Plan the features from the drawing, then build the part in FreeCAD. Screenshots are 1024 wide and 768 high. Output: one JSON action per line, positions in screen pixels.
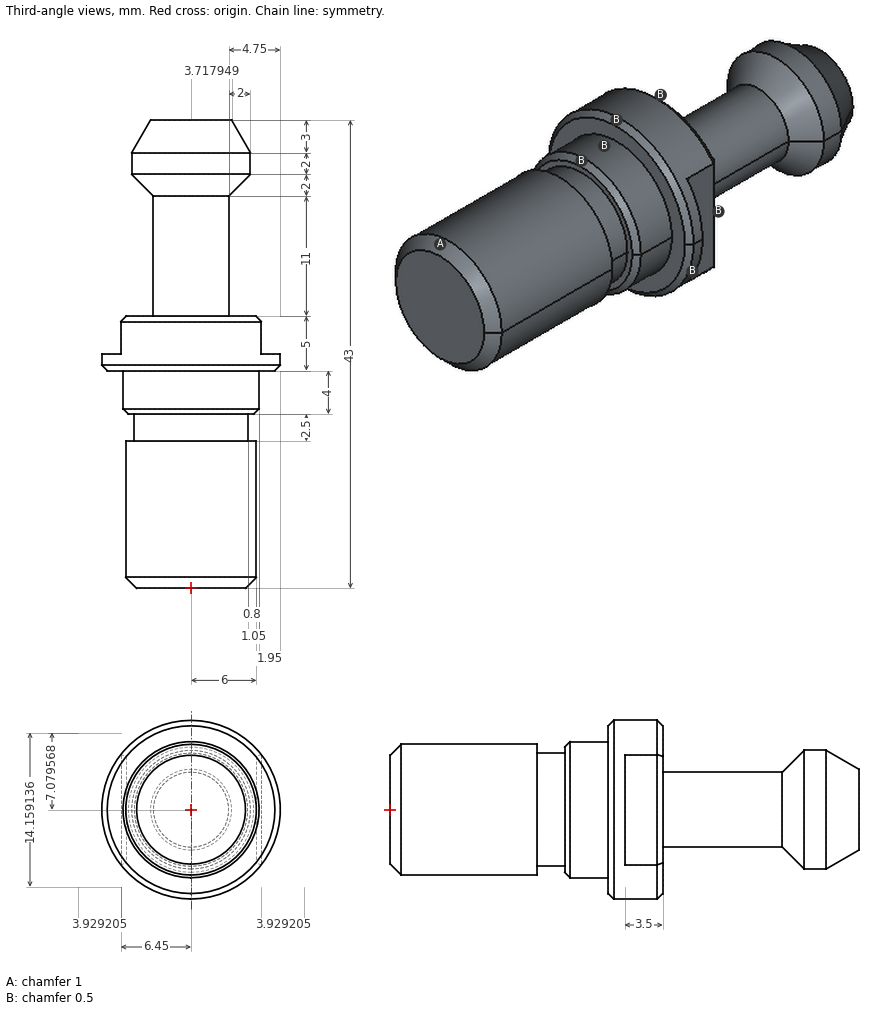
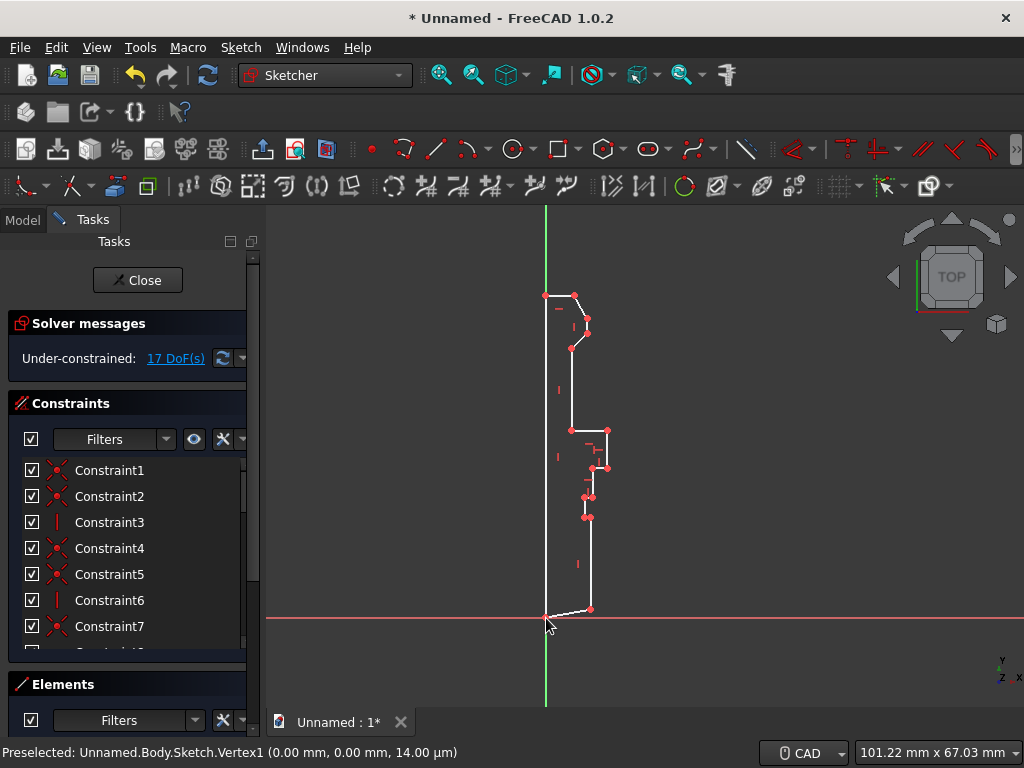
{"action": "left_click", "coordinate": [559, 615]}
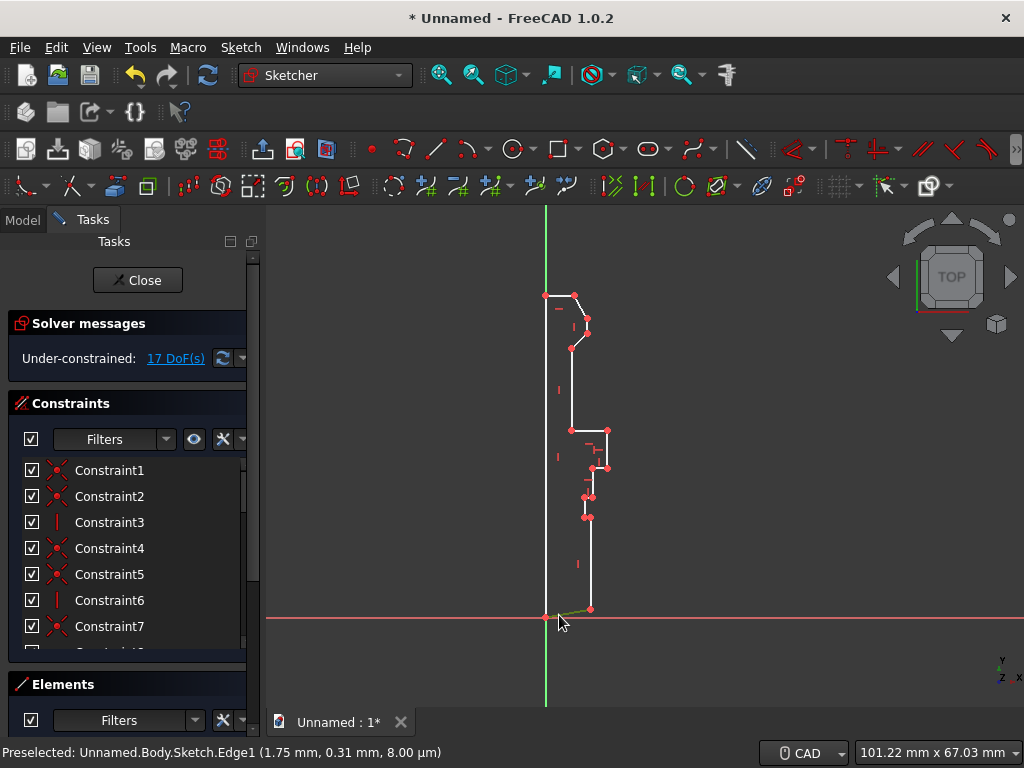
{"action": "key", "text": "h"}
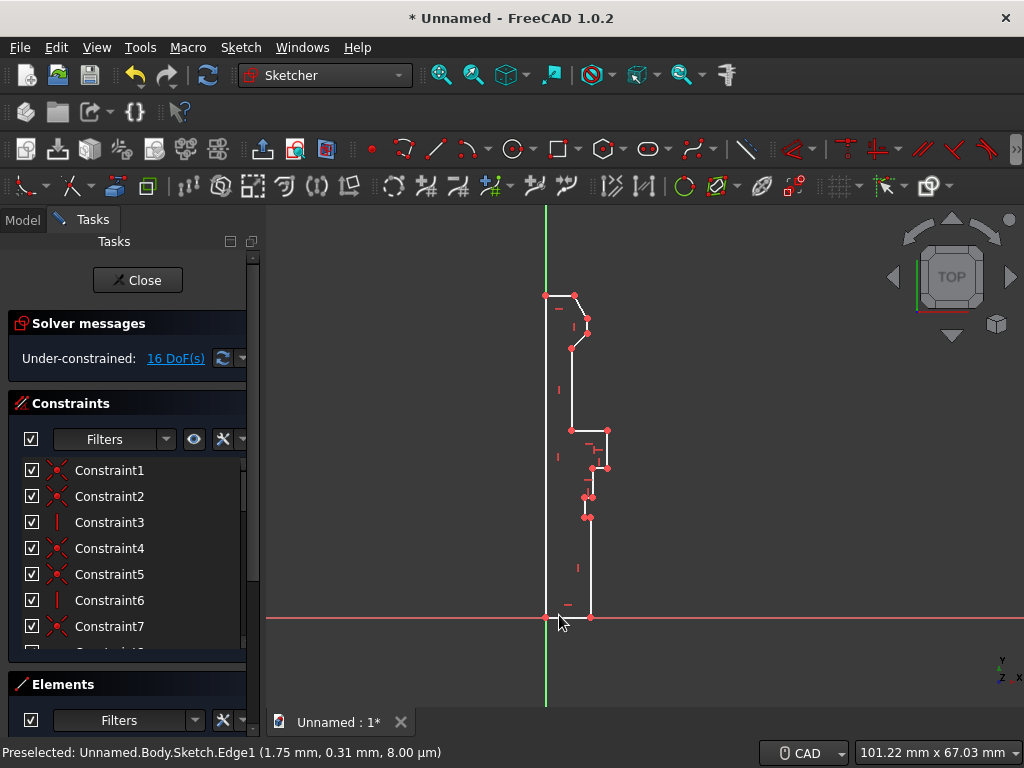
{"action": "scroll", "coordinate": [588, 517], "scroll_direction": "up", "scroll_amount": 8}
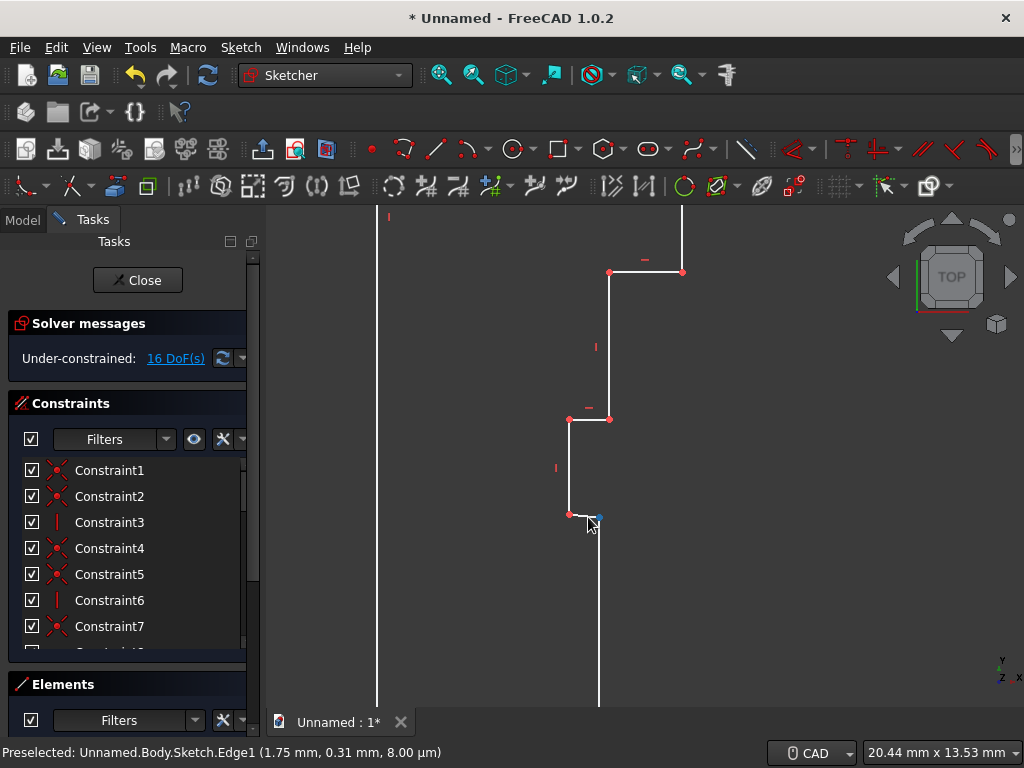
{"action": "left_click", "coordinate": [584, 516]}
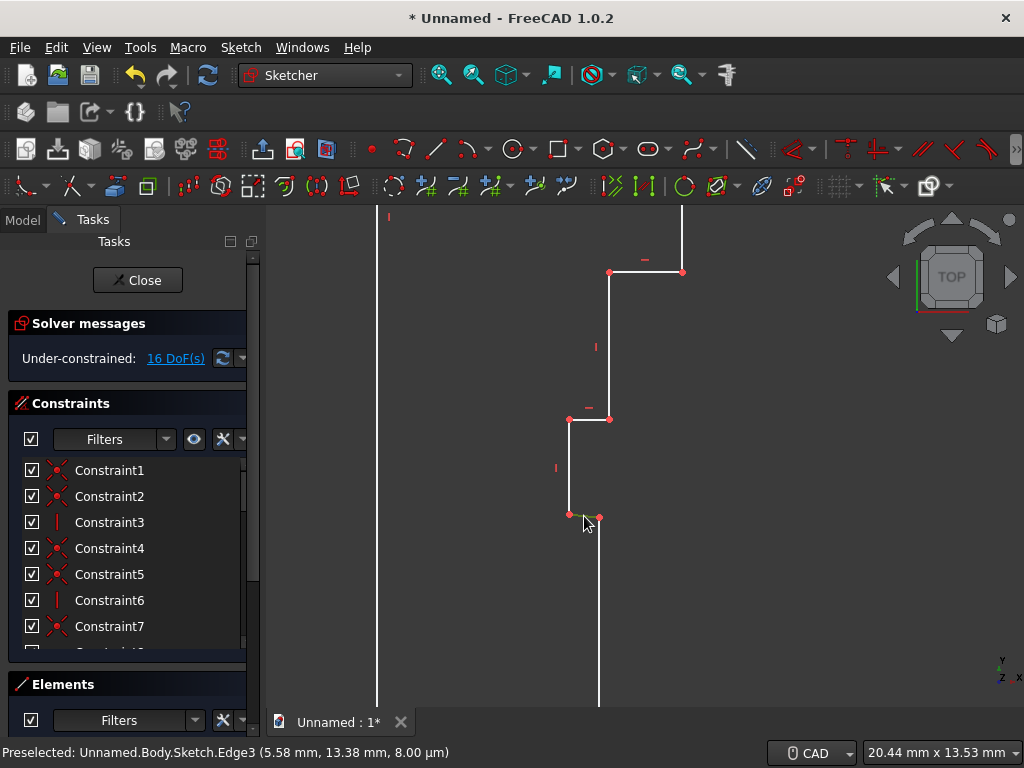
{"action": "left_click", "coordinate": [900, 150]}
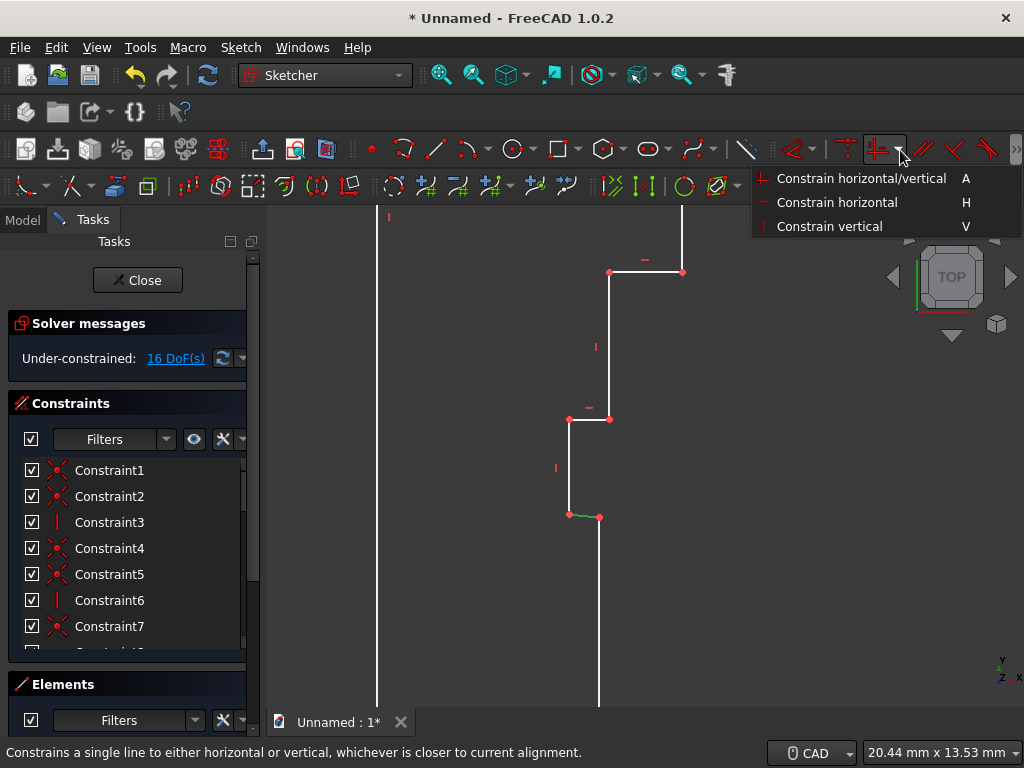
{"action": "left_click", "coordinate": [887, 202]}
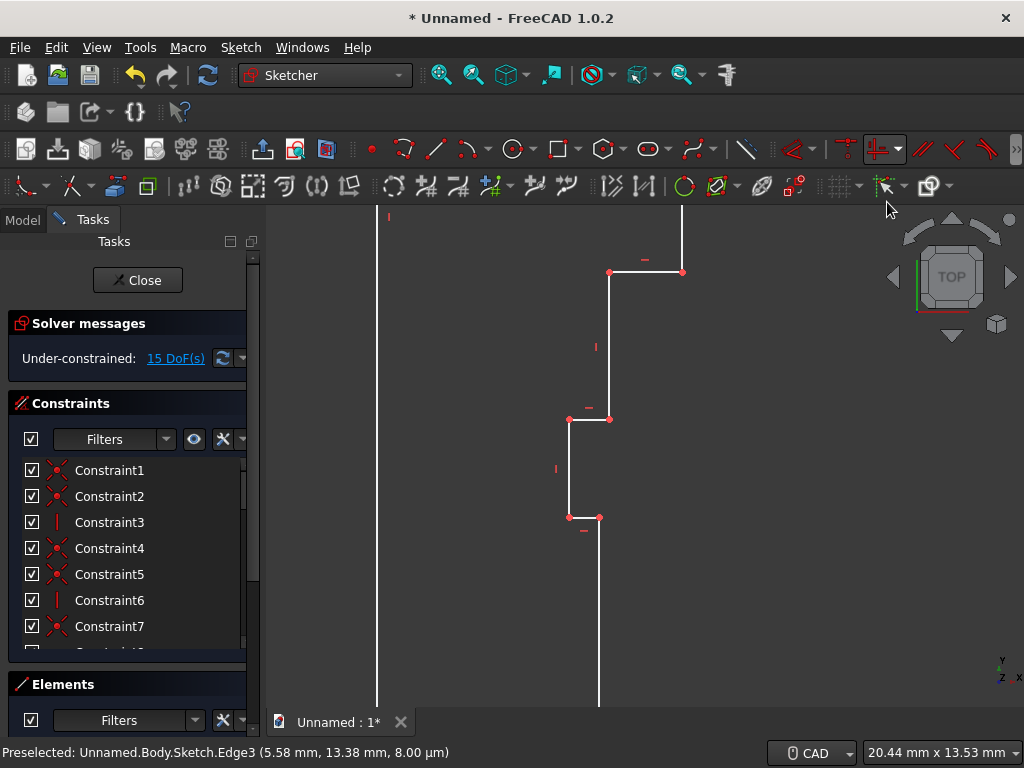
{"action": "left_click", "coordinate": [792, 150]}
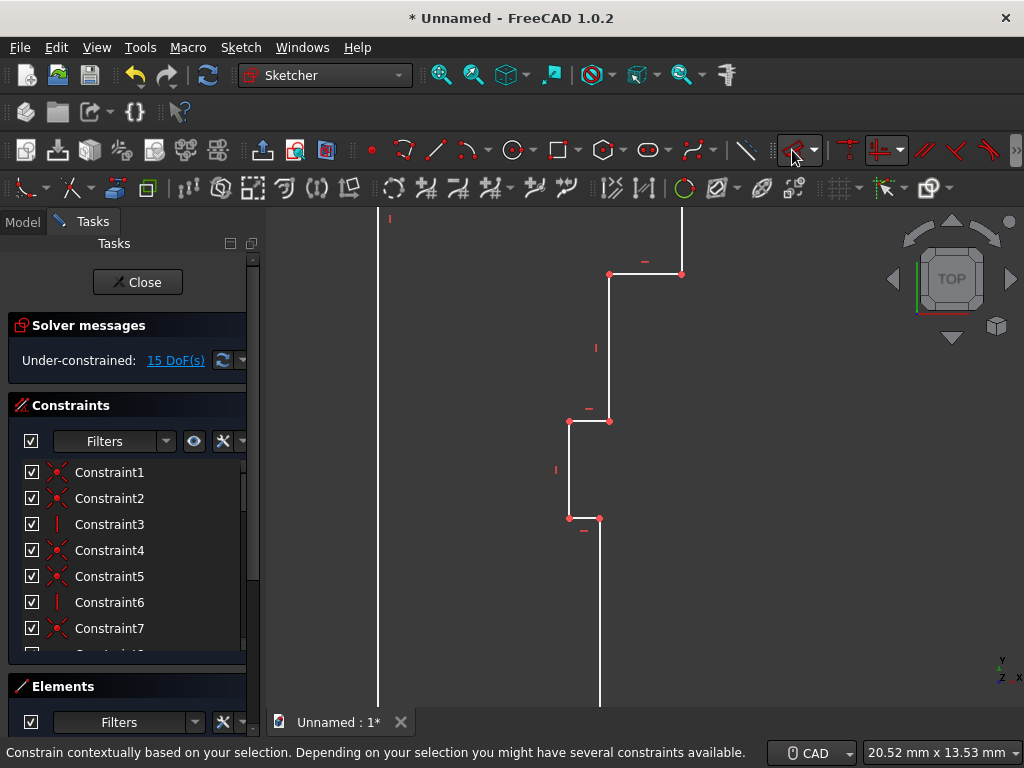
{"action": "scroll", "coordinate": [588, 518], "scroll_direction": "down", "scroll_amount": 8}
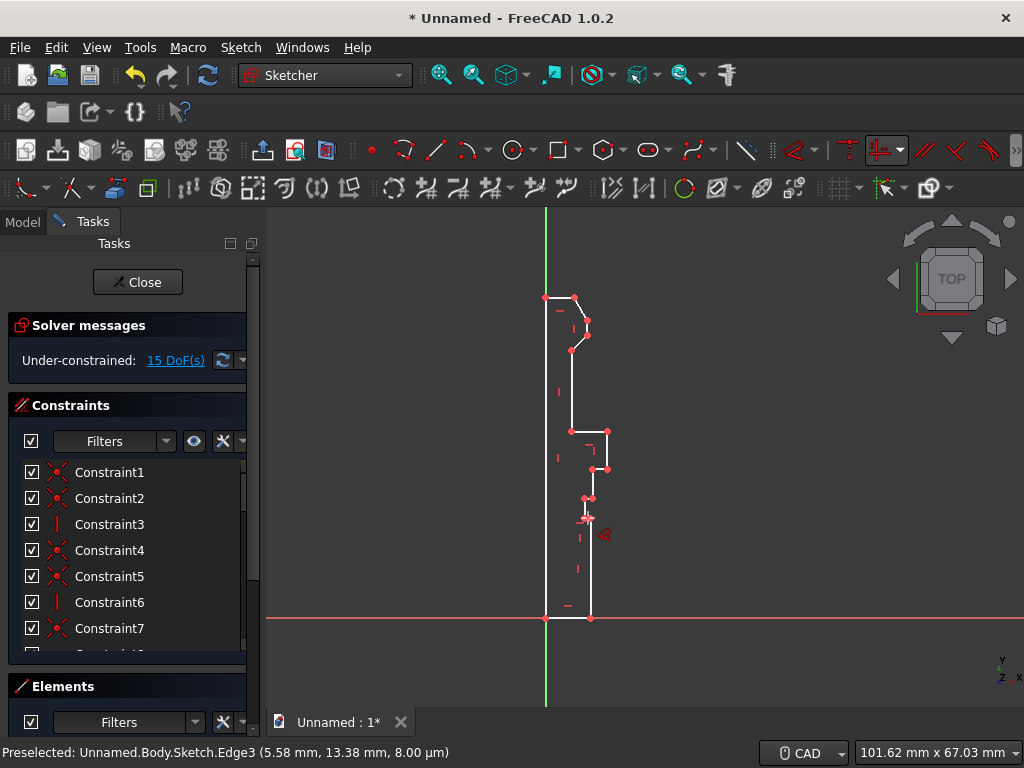
{"action": "left_click", "coordinate": [559, 618]}
{"action": "left_click", "coordinate": [568, 652]}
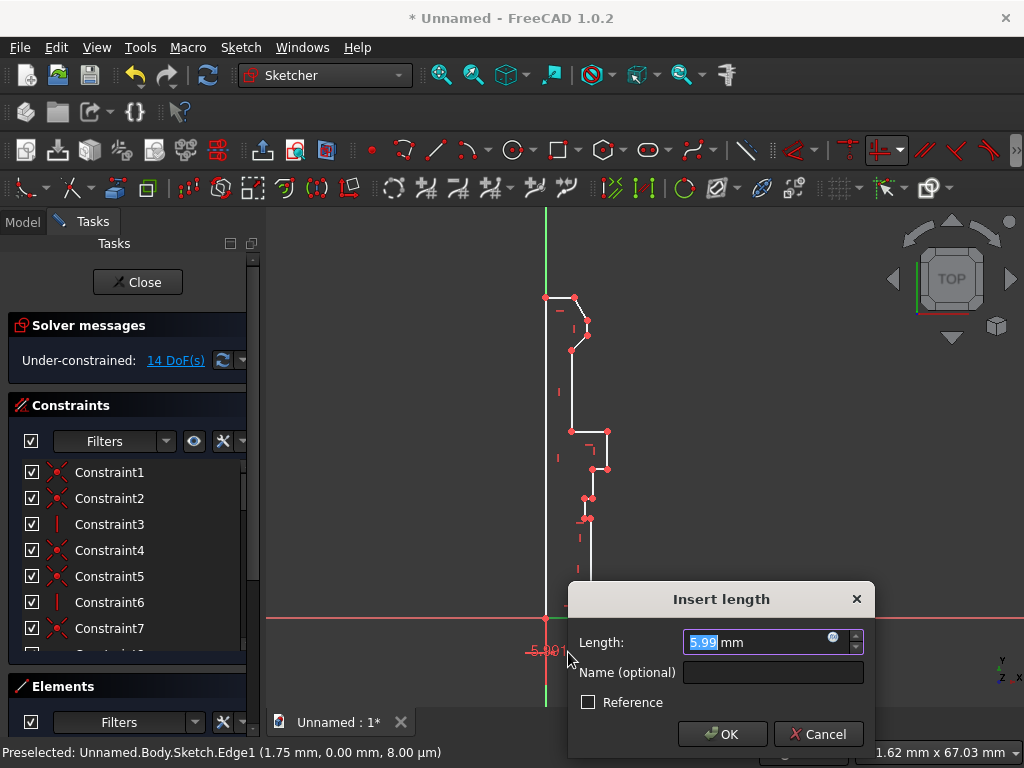
{"action": "type", "text": "6"}
{"action": "key", "text": "Return"}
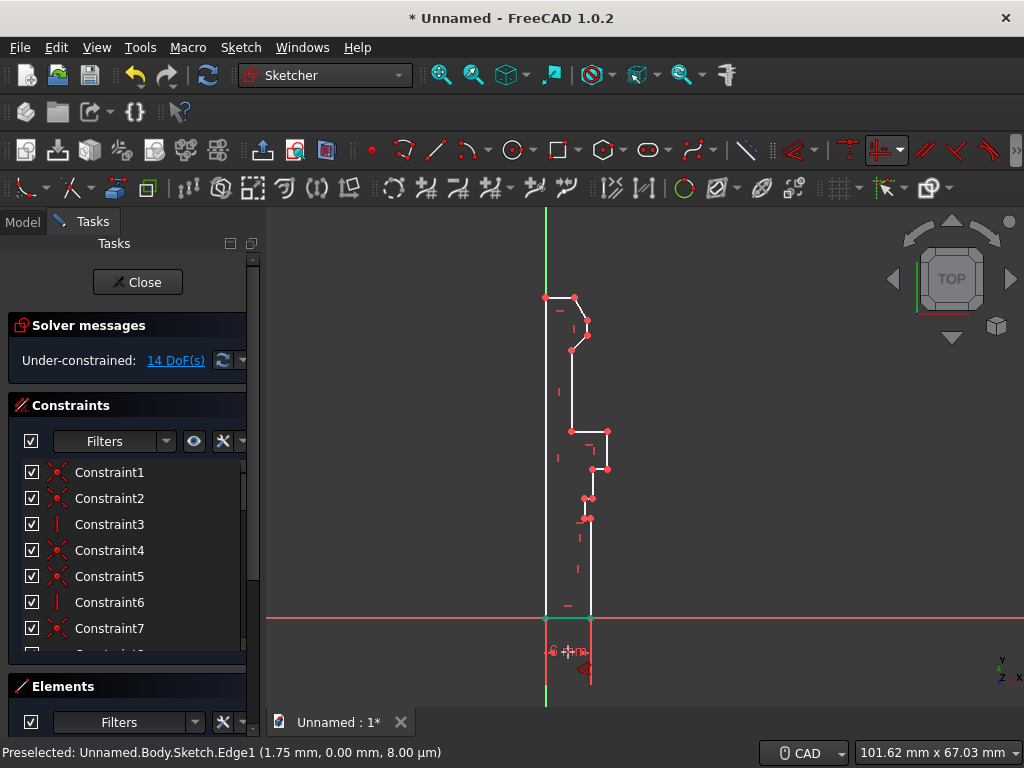
{"action": "scroll", "coordinate": [593, 487], "scroll_direction": "up", "scroll_amount": 2}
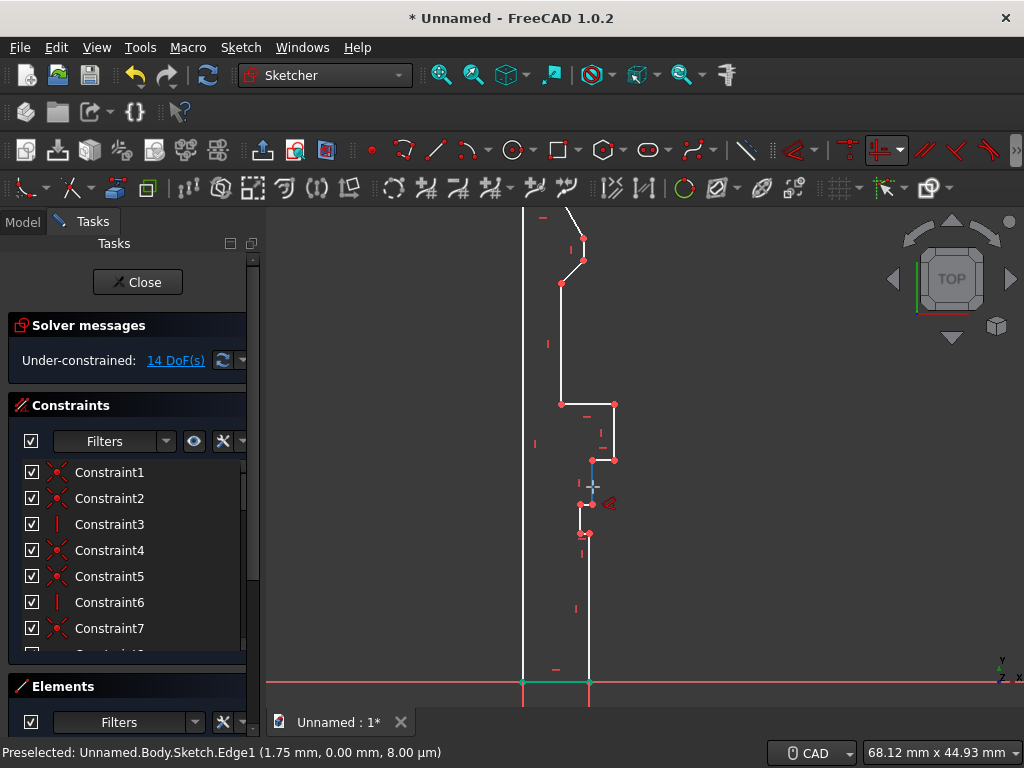
{"action": "left_click", "coordinate": [592, 487]}
{"action": "left_click", "coordinate": [626, 482]}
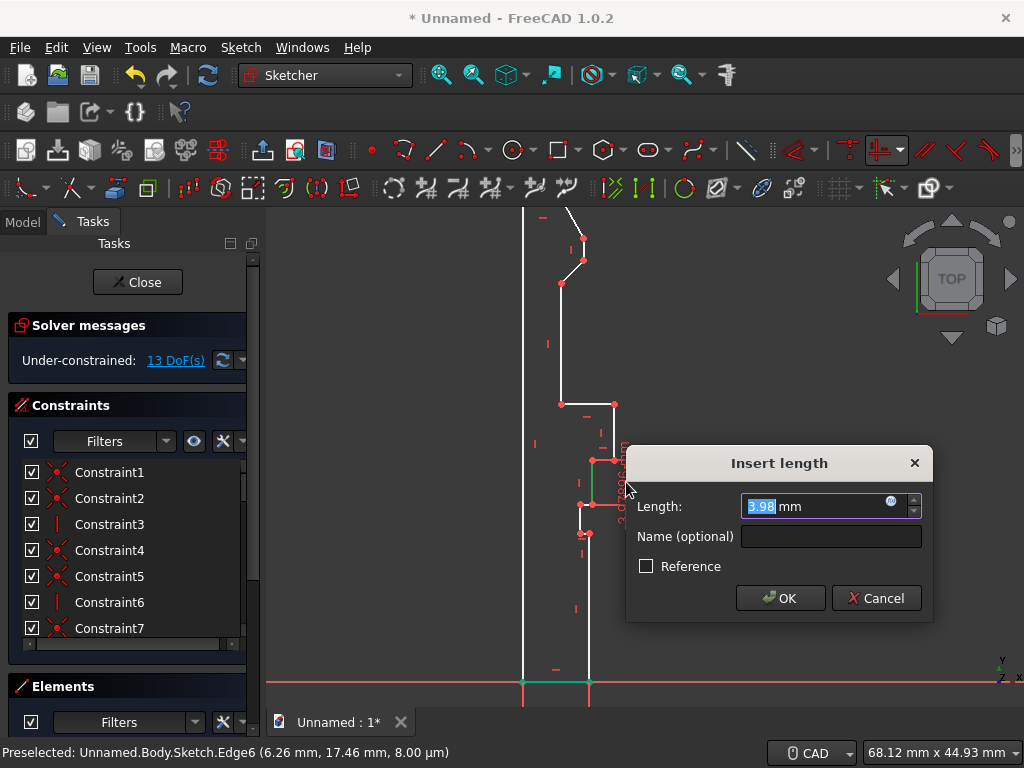
{"action": "type", "text": "4"}
{"action": "key", "text": "Return"}